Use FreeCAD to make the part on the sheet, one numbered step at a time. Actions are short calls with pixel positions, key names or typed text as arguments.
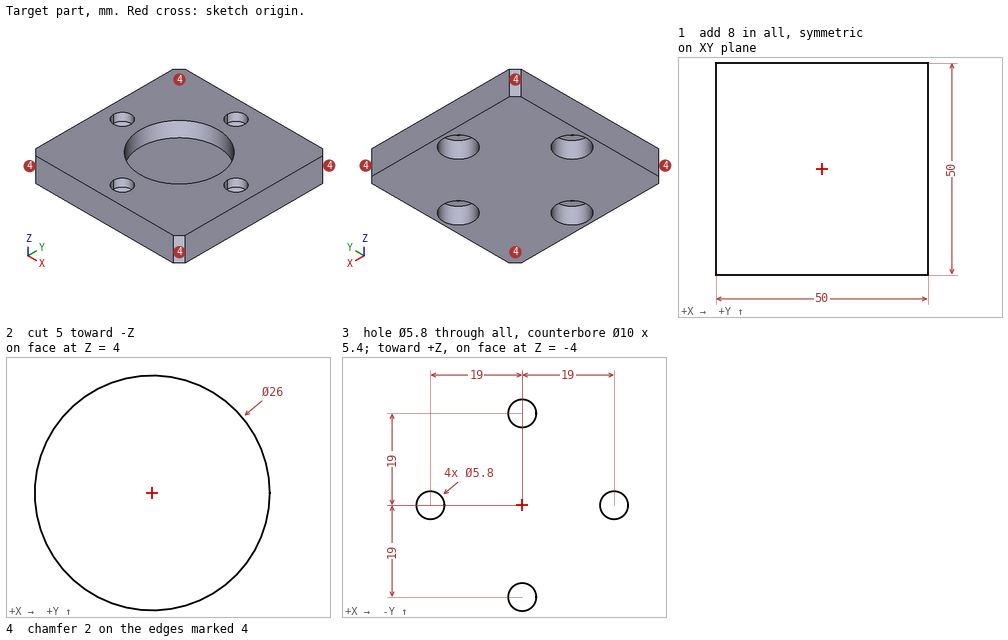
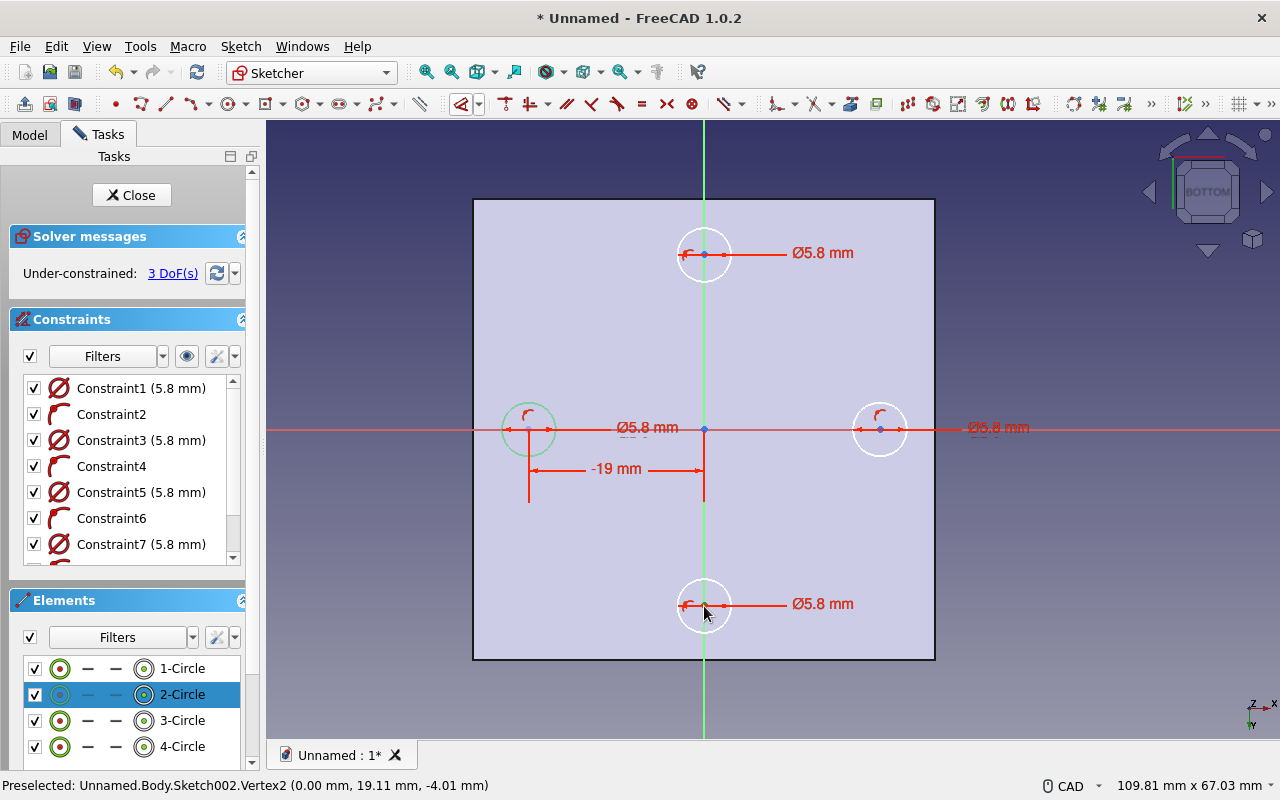
key(i)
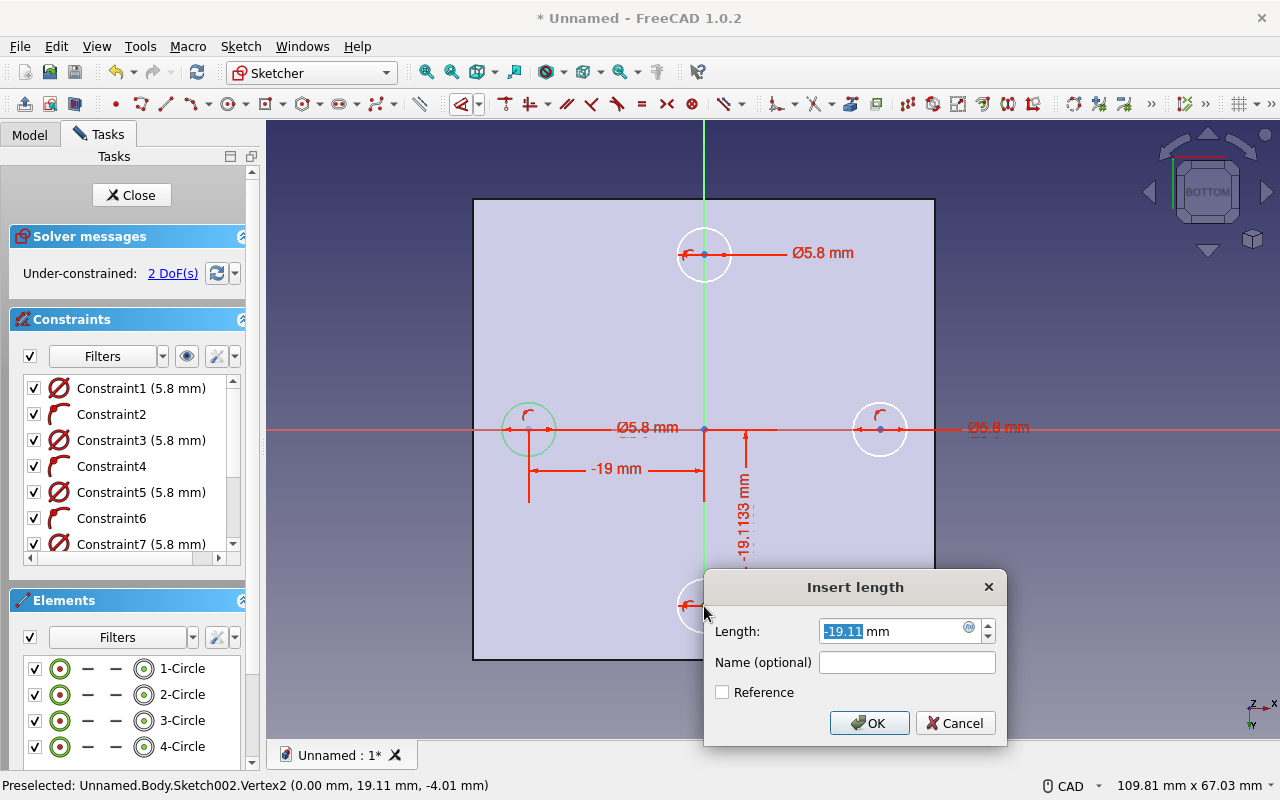
text(-19)
key(Return)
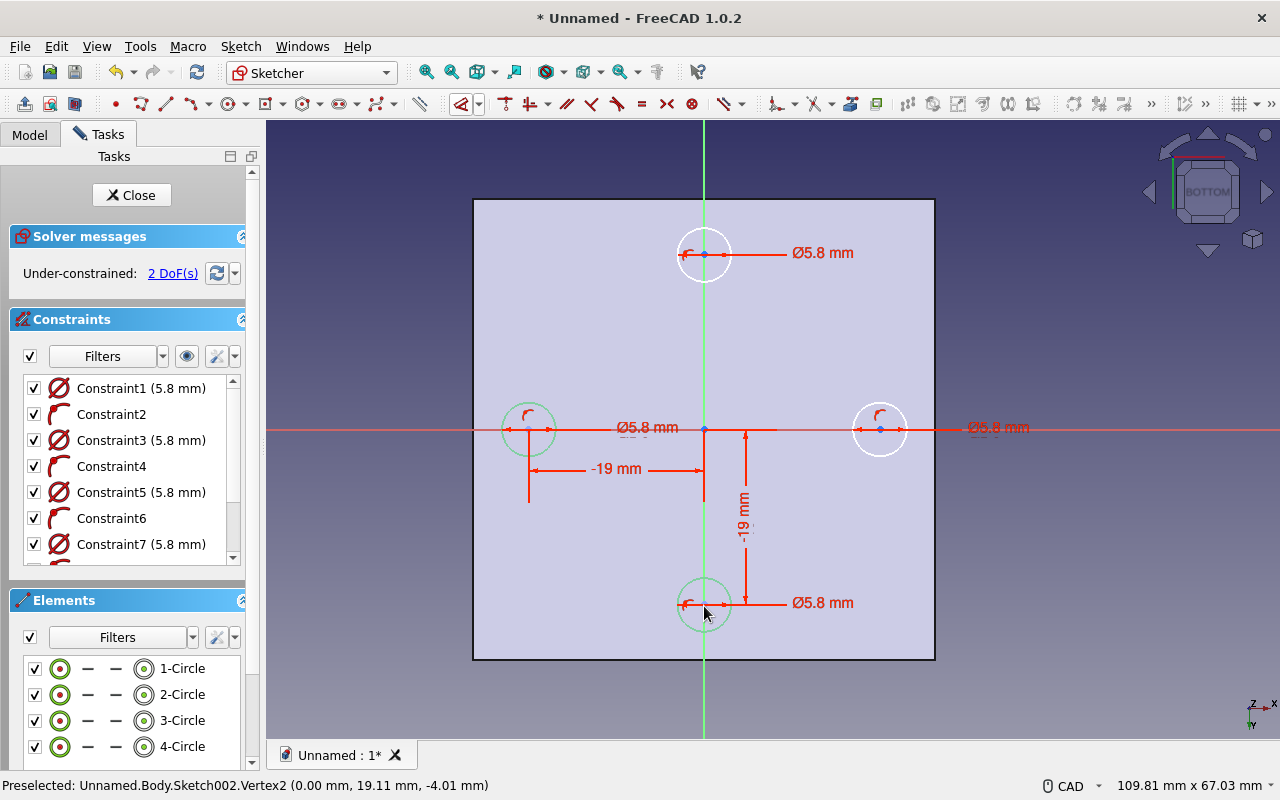
click(880, 430)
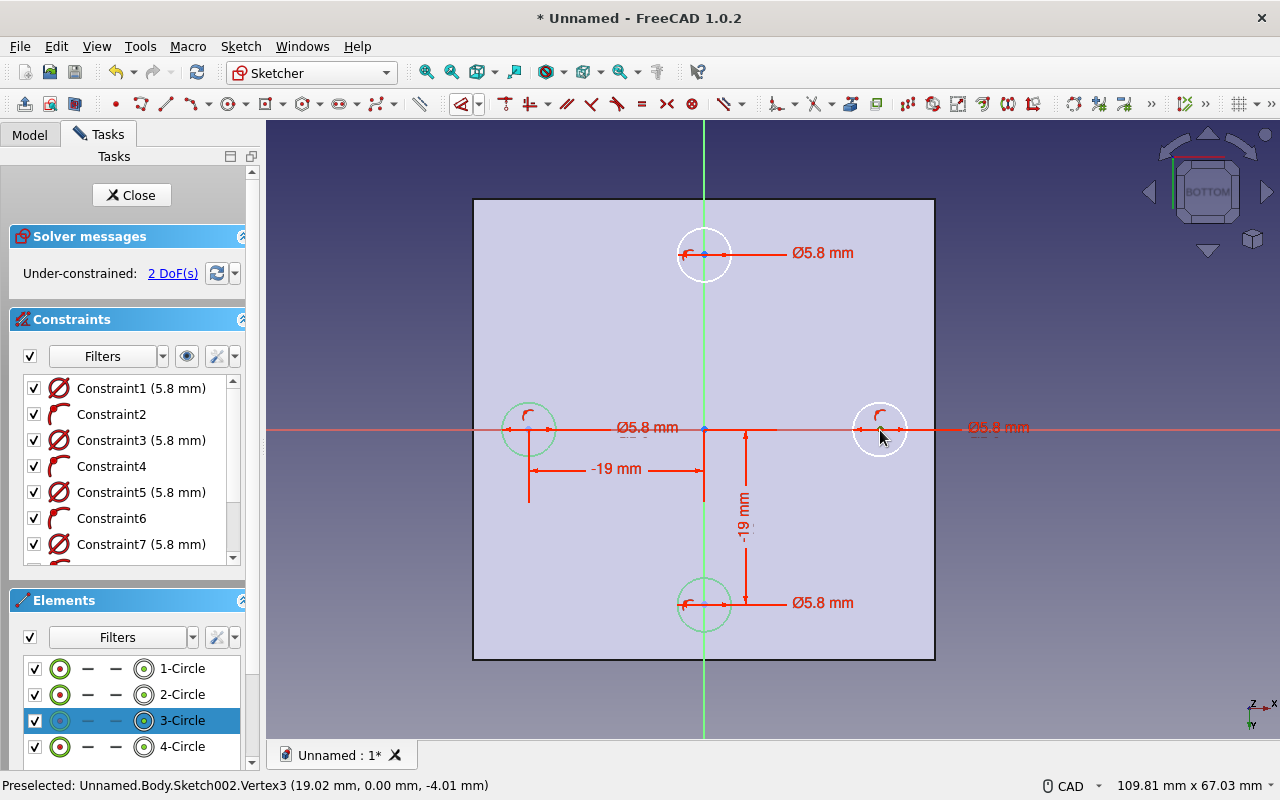
key(l)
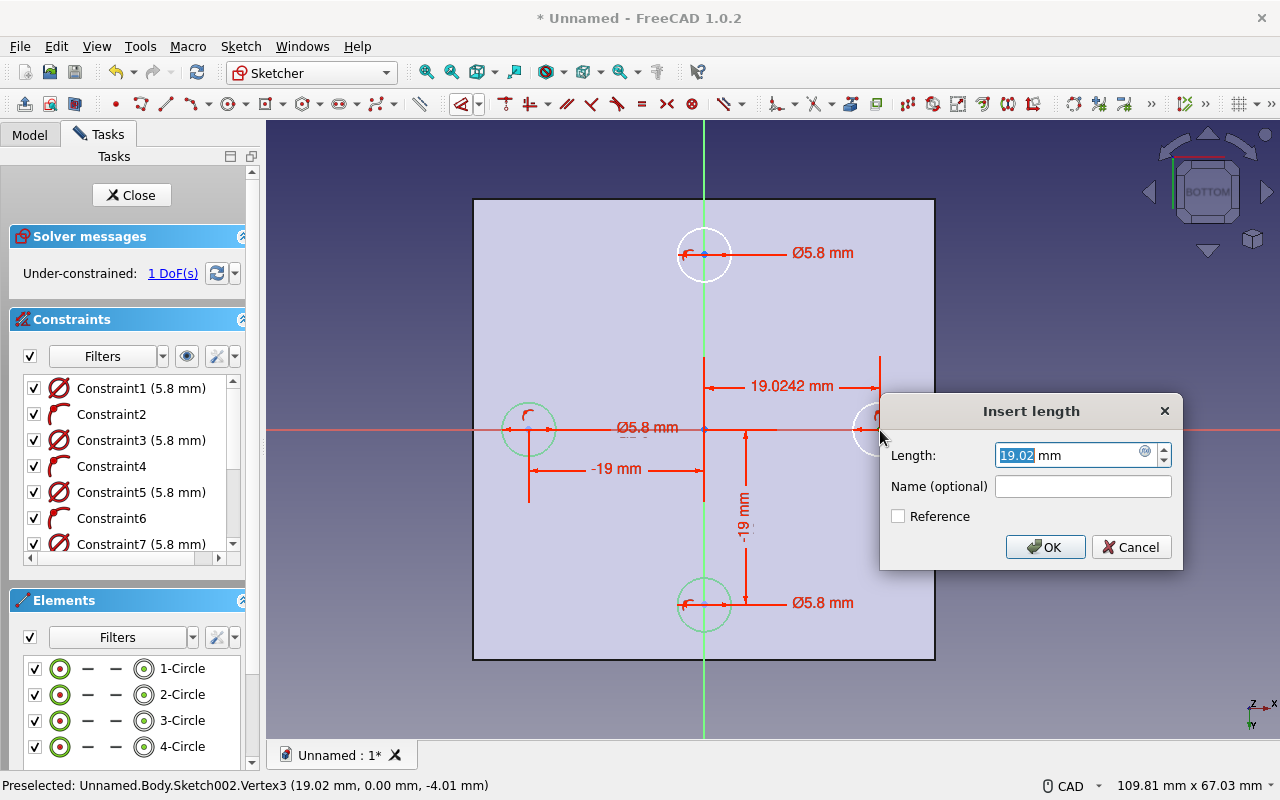
text(19)
key(Return)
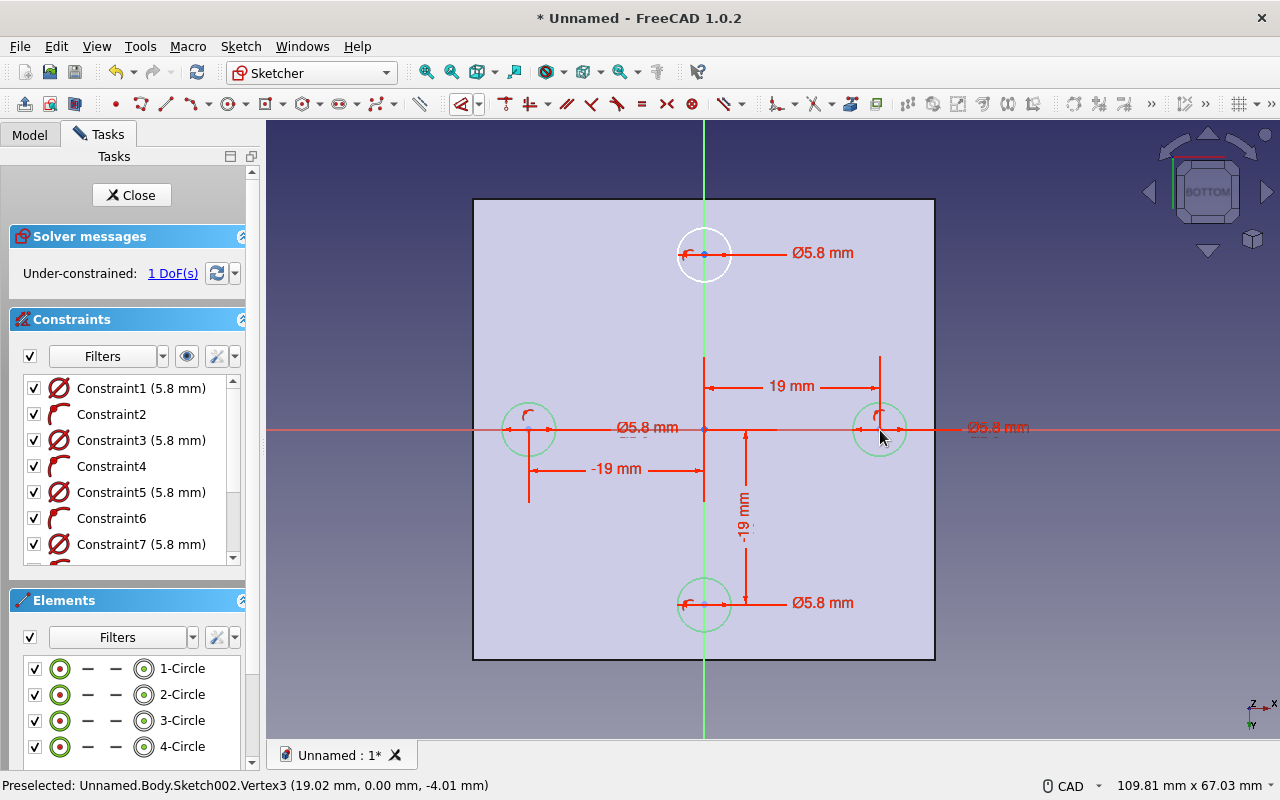
click(704, 255)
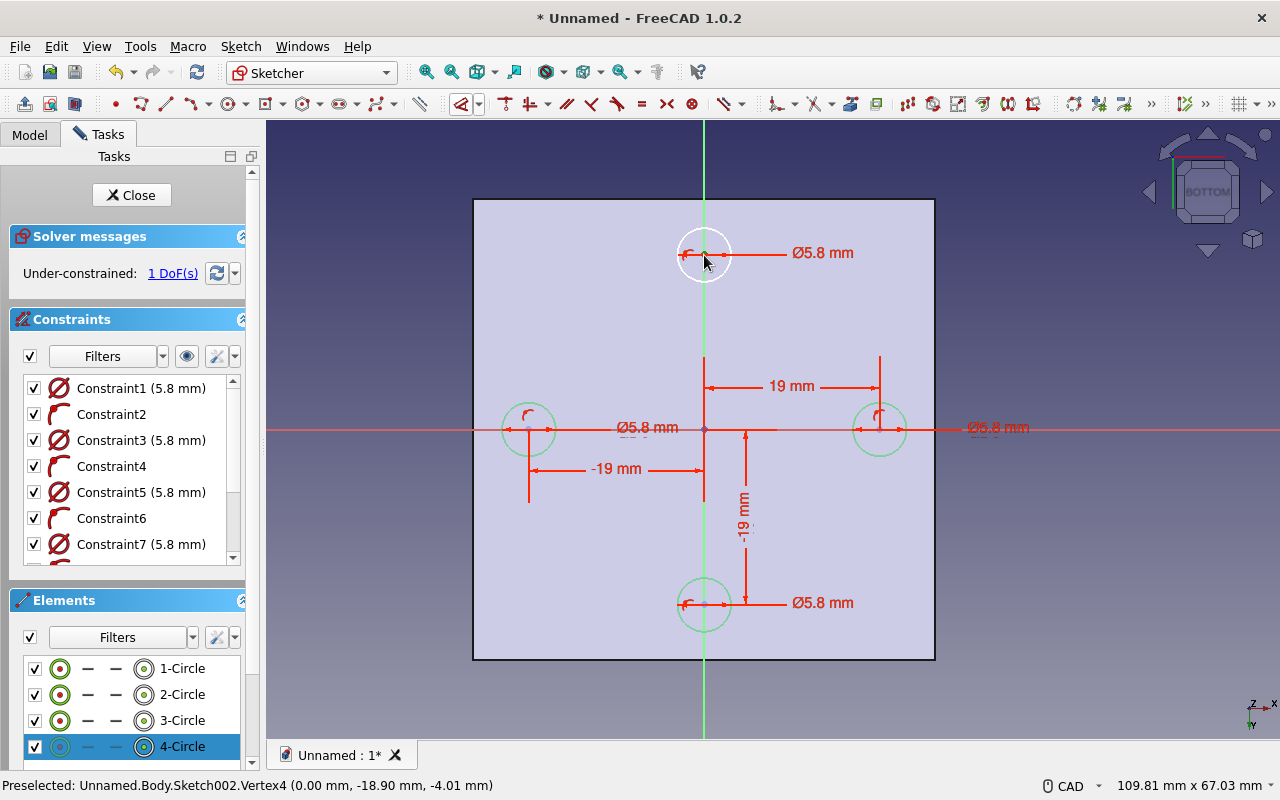
key(i)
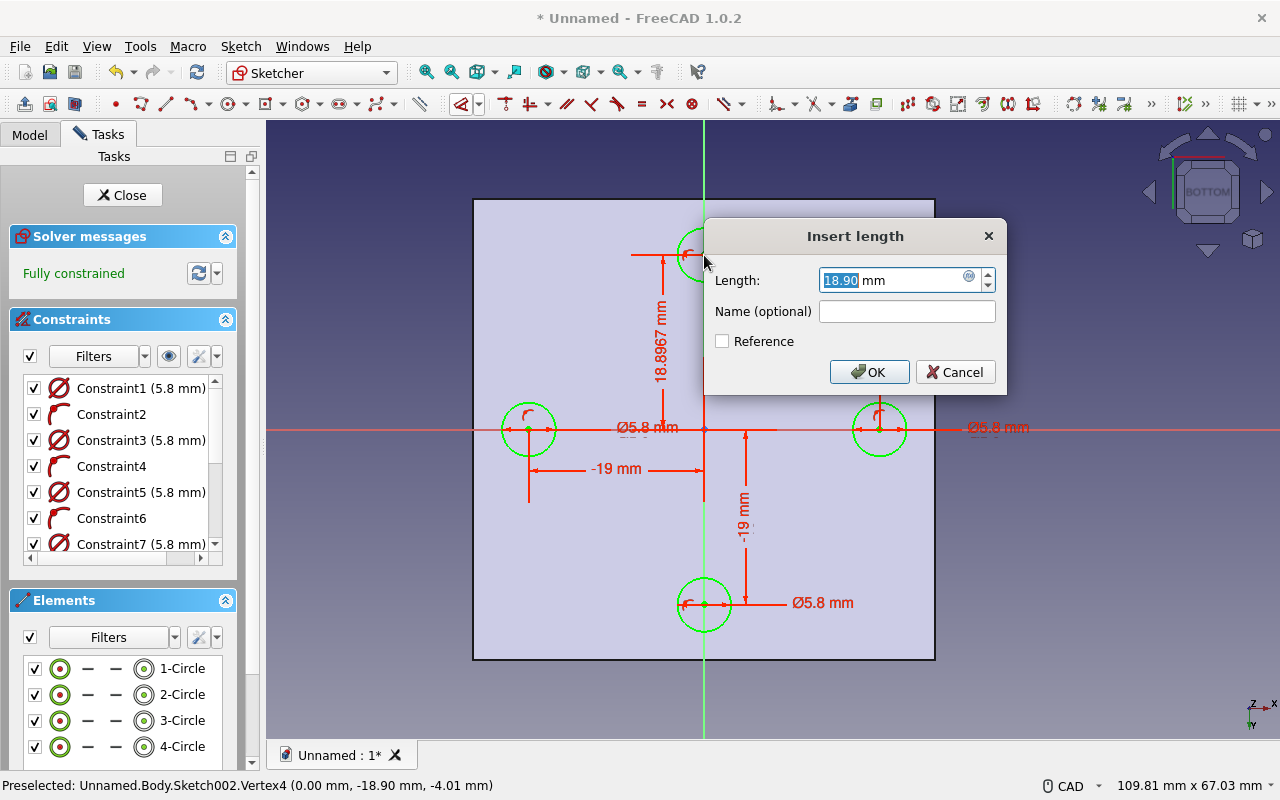
text(19)
key(Return)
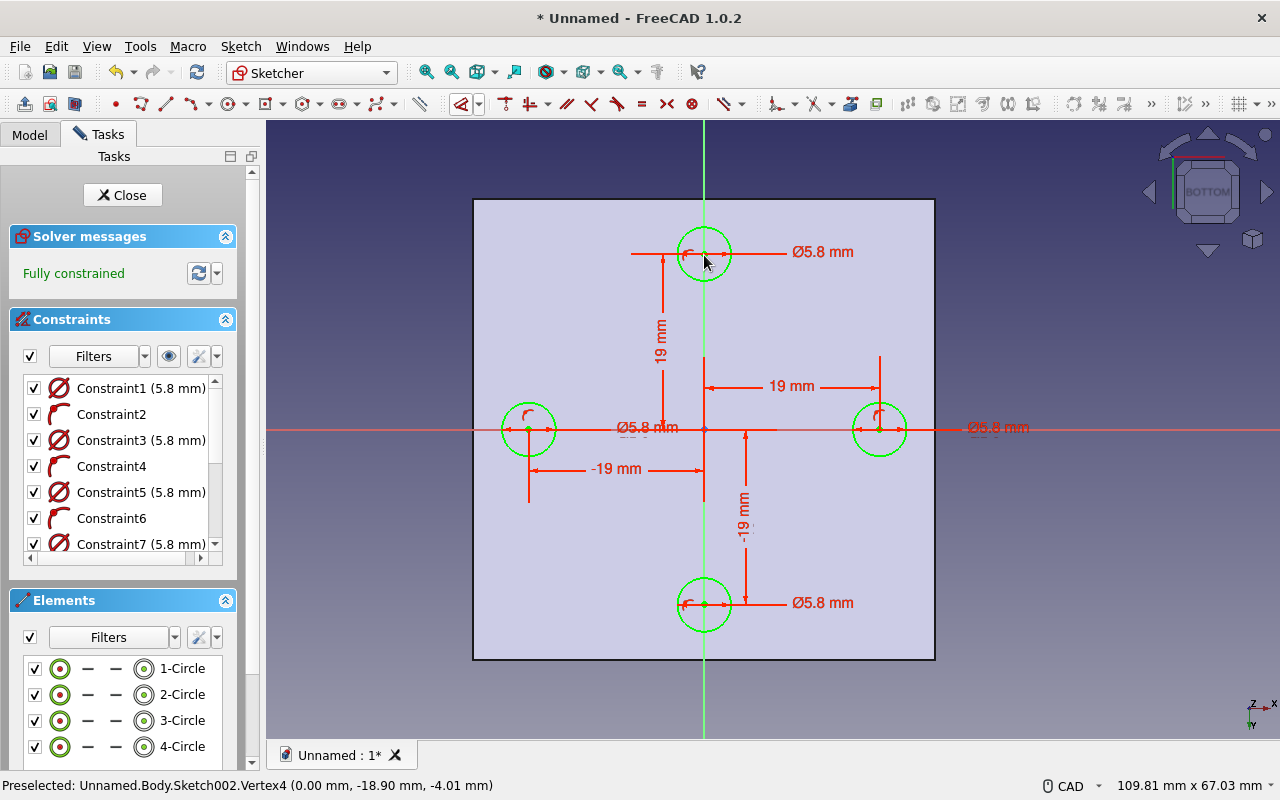
click(123, 195)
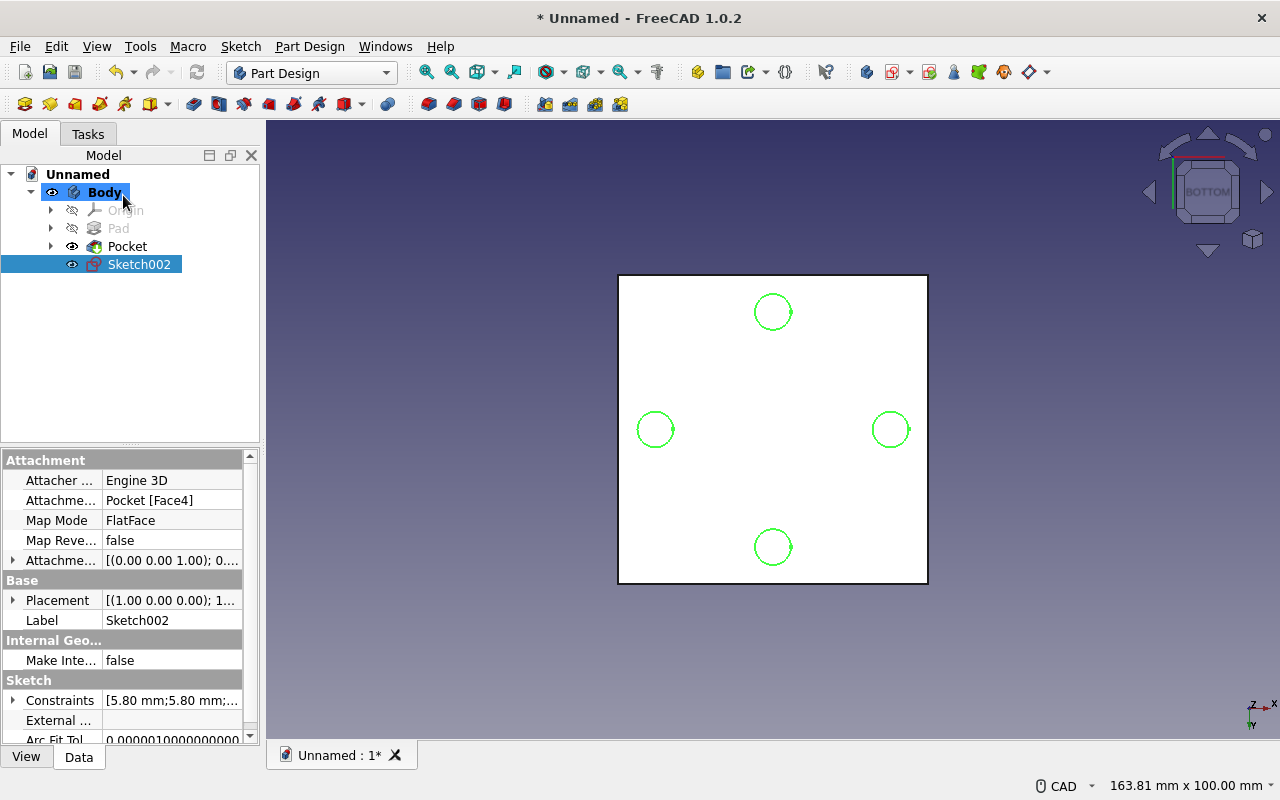
click(219, 104)